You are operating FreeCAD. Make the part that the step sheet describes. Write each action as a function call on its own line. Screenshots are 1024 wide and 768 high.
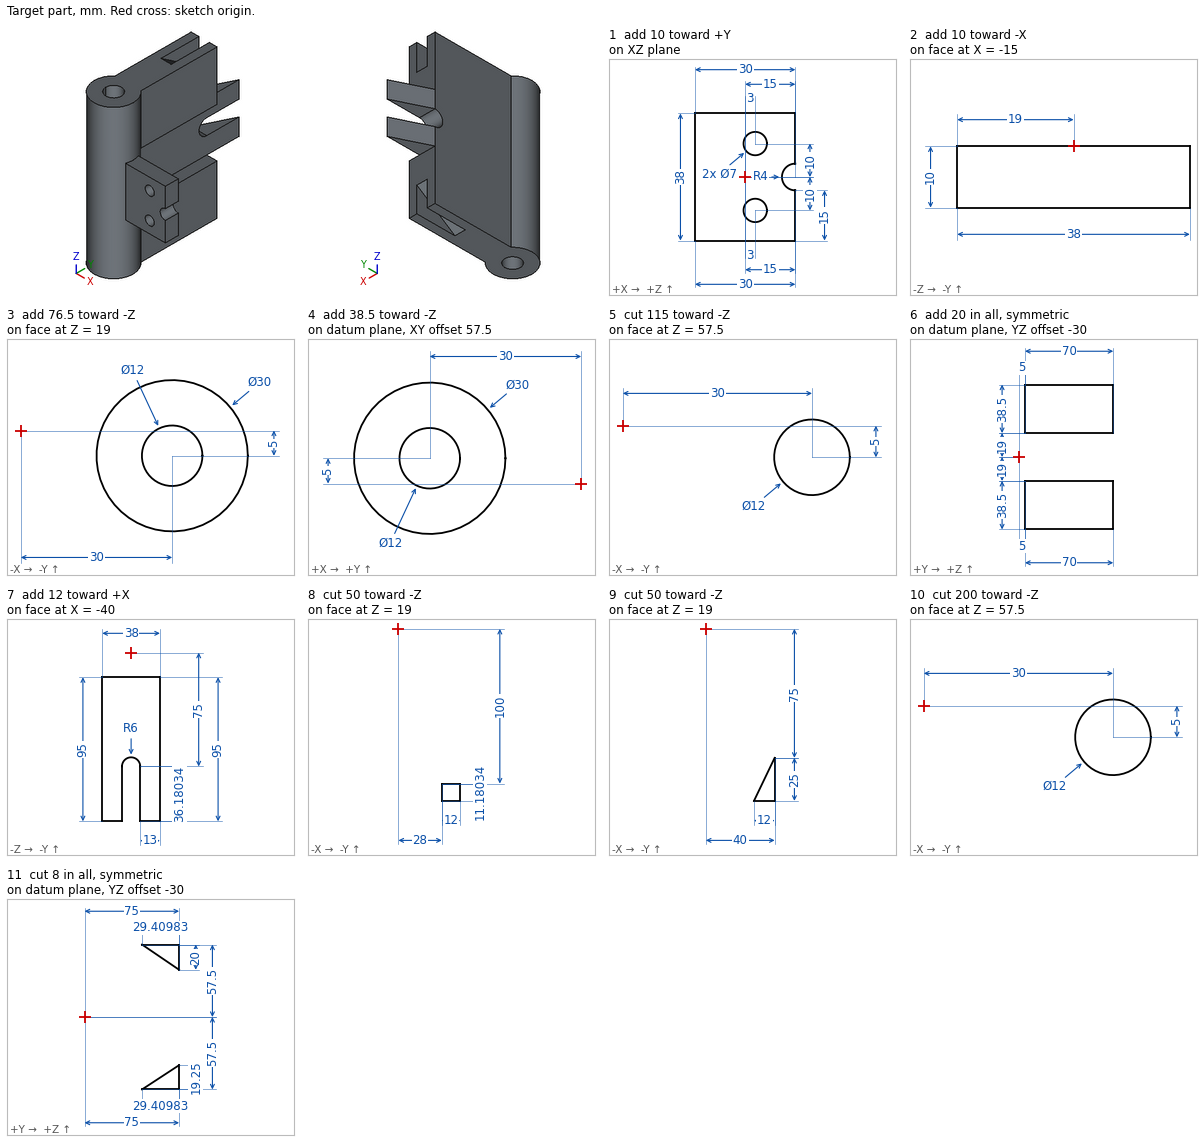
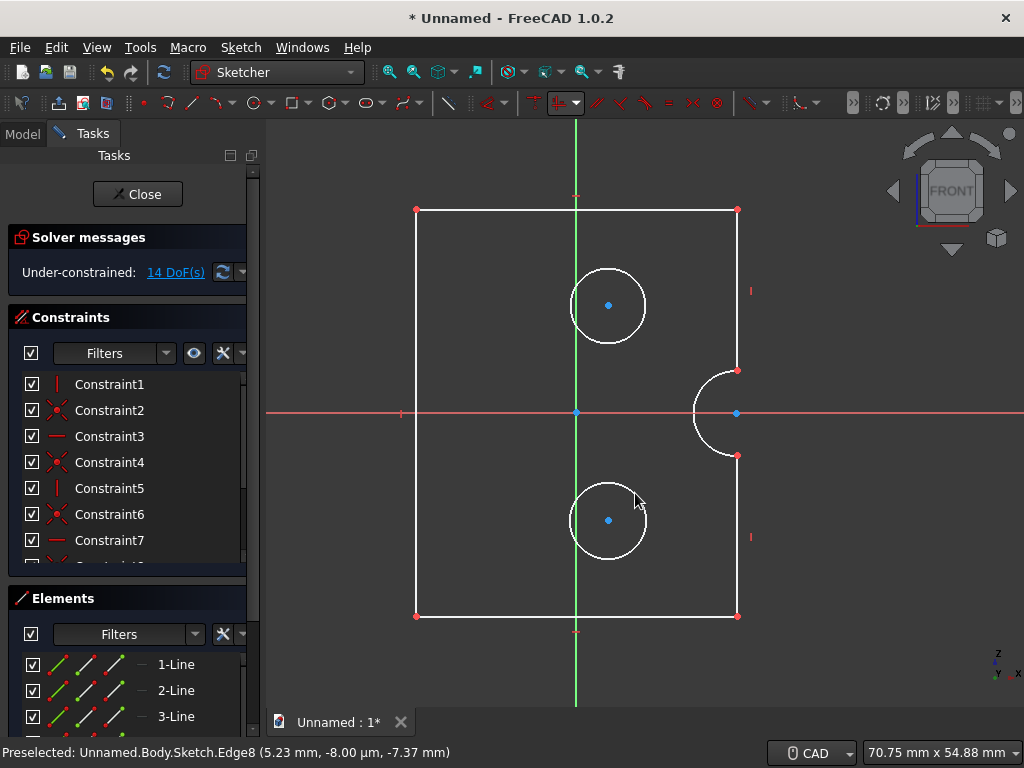
click(634, 279)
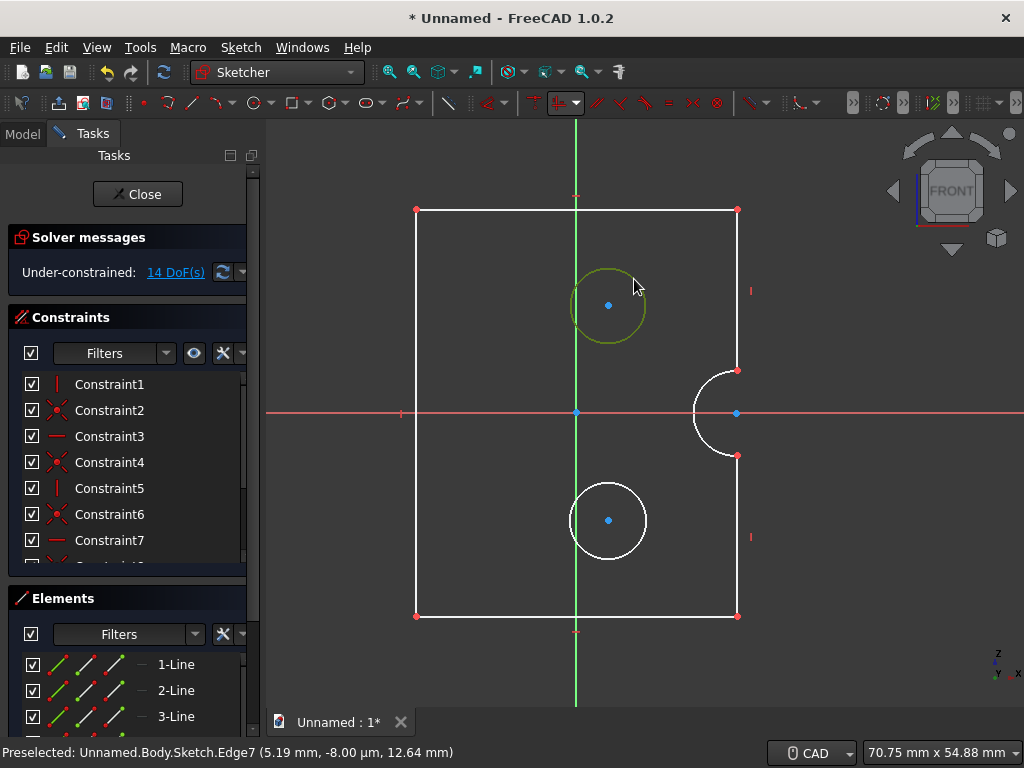
click(635, 494)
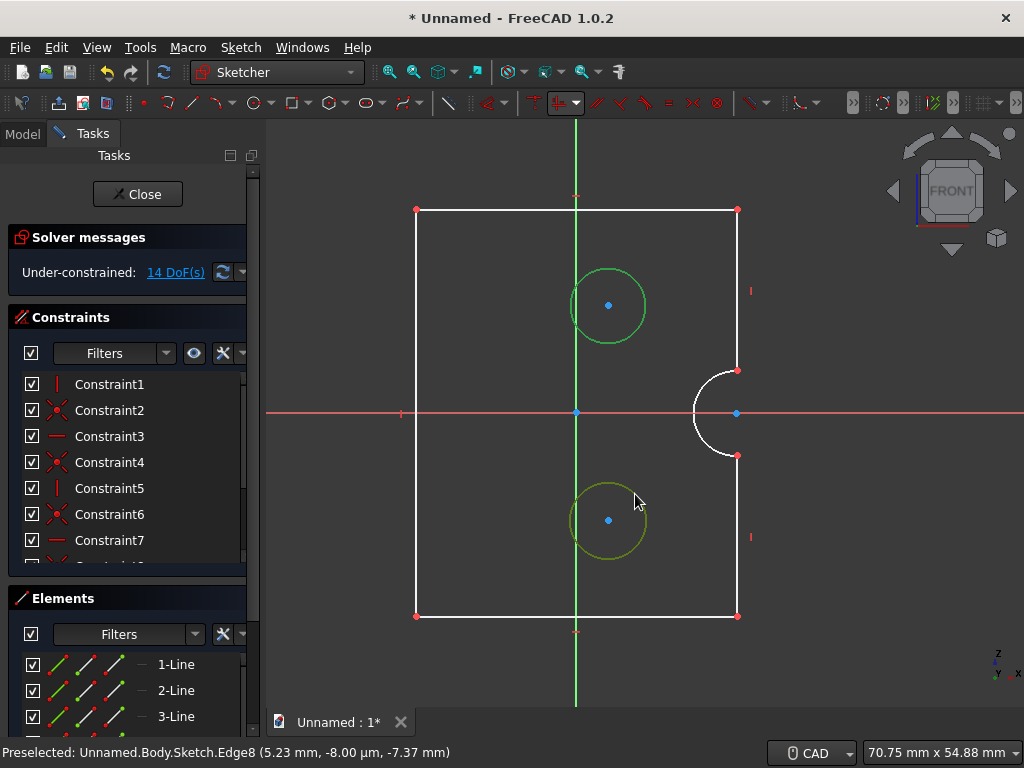
key(e)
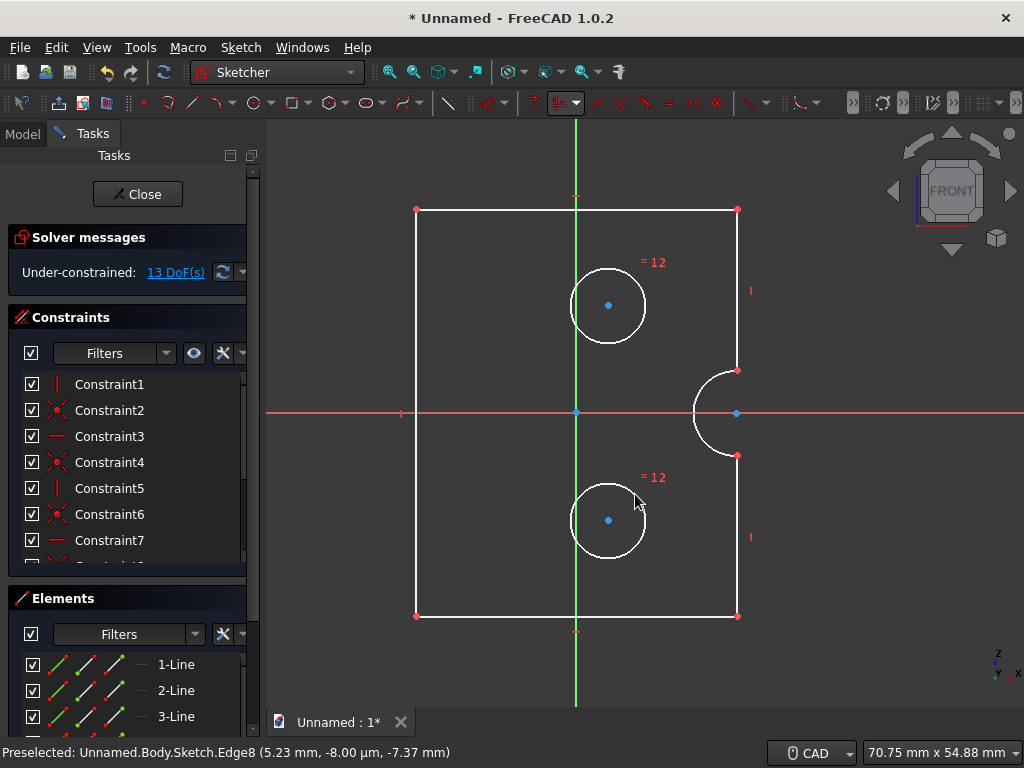
click(736, 414)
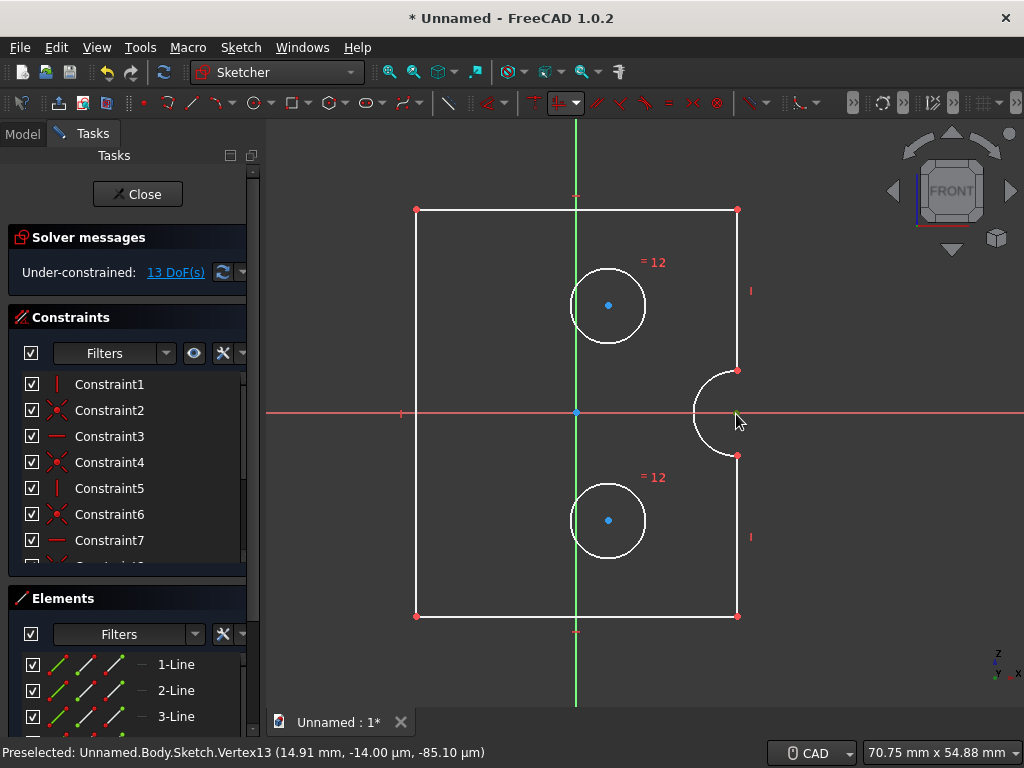
click(334, 413)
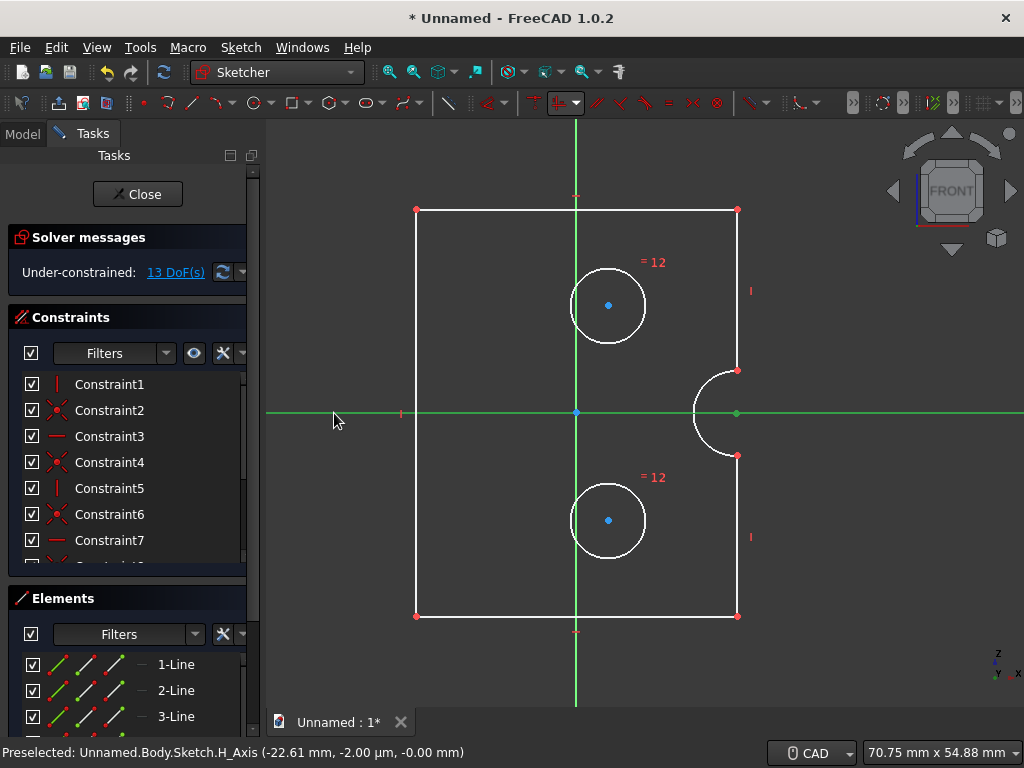
click(534, 104)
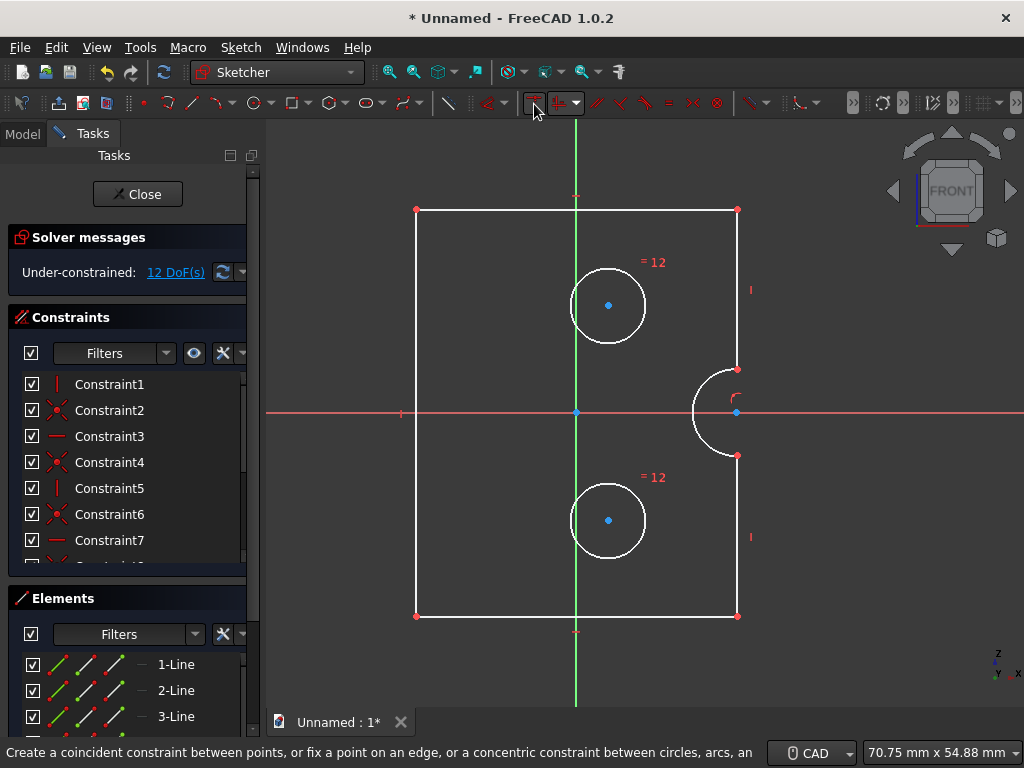
click(701, 387)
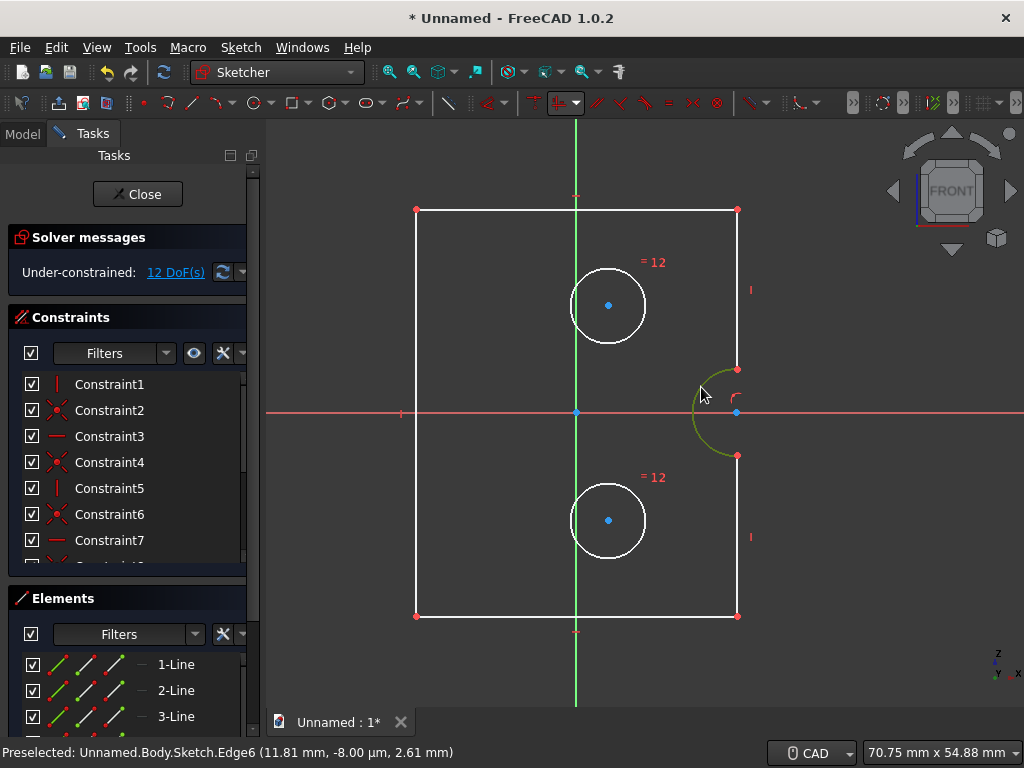
key(k)
key(r)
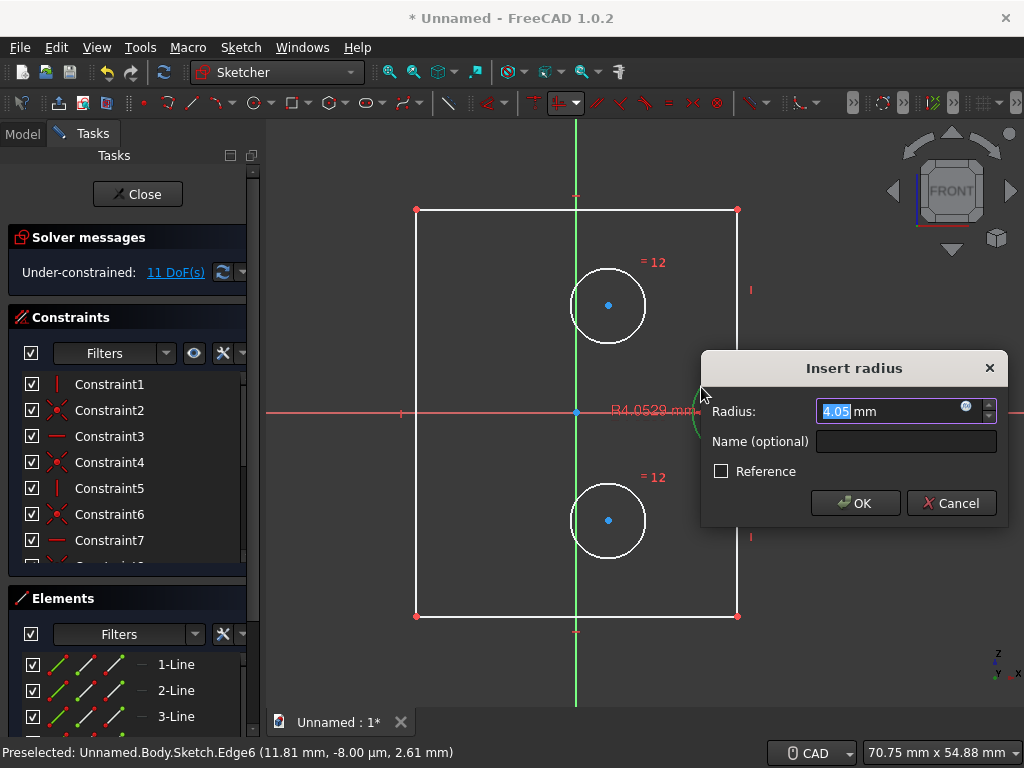
text(4)
key(Return)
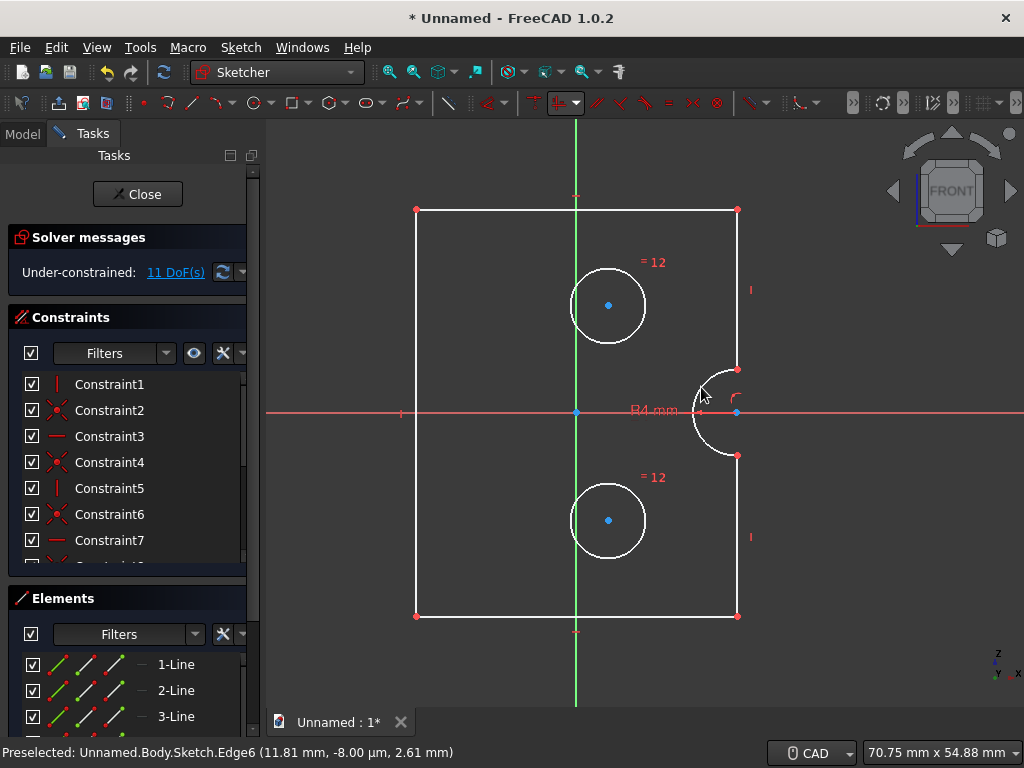
click(634, 279)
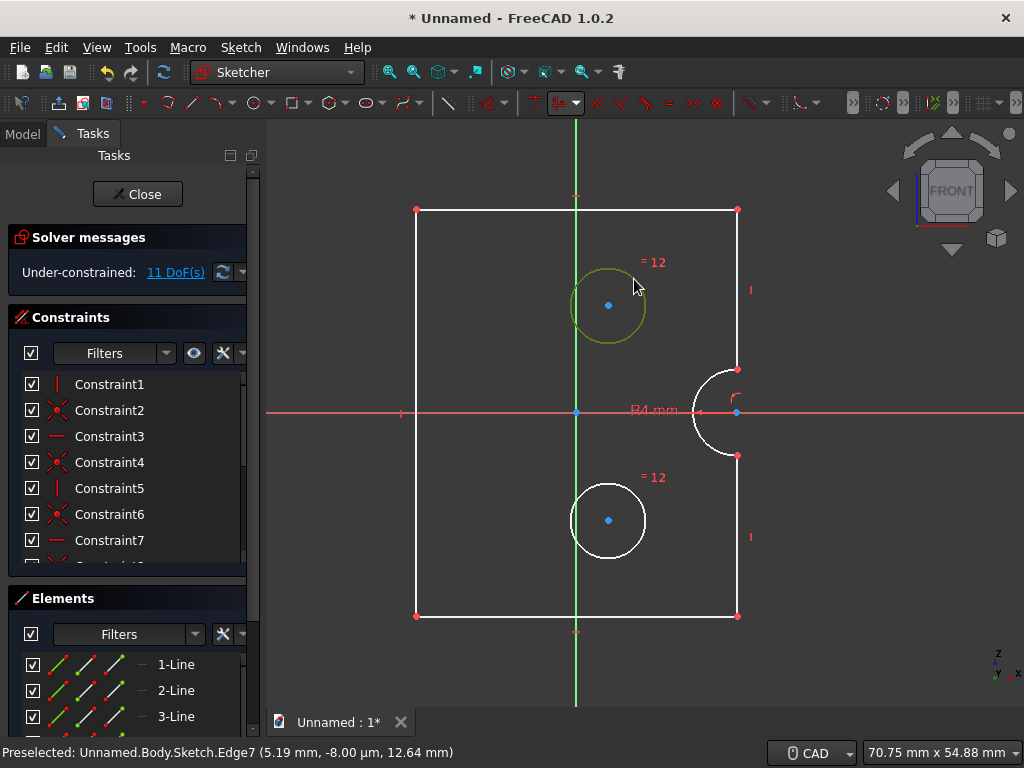
key(k)
key(o)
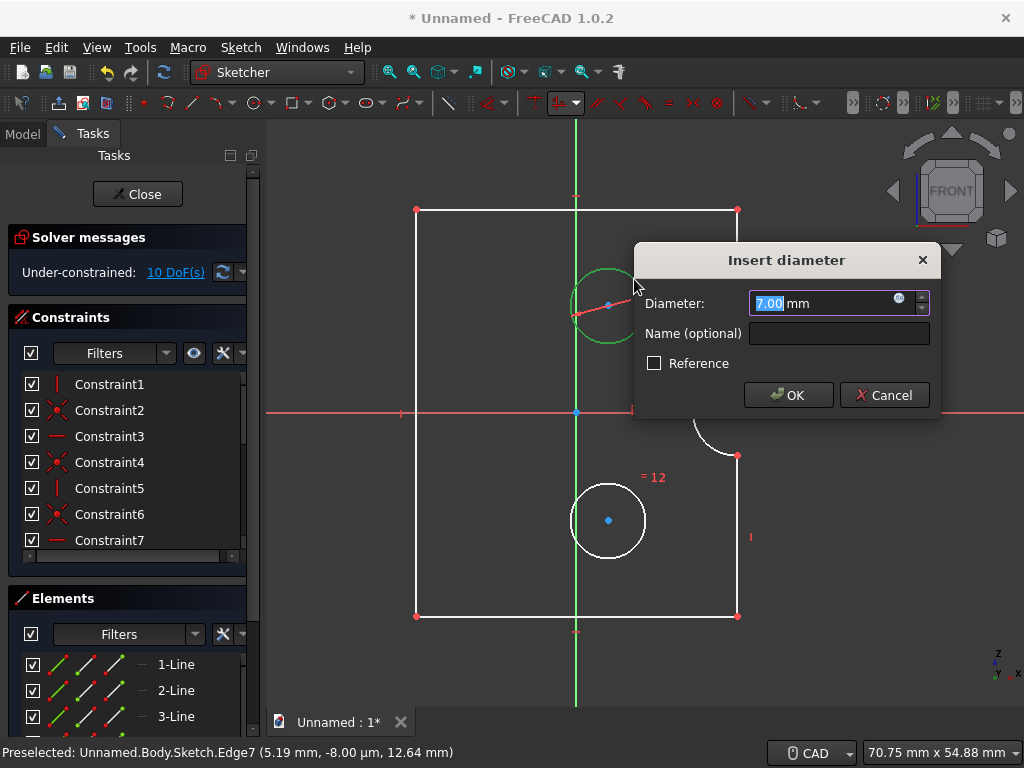
text(7)
key(Return)